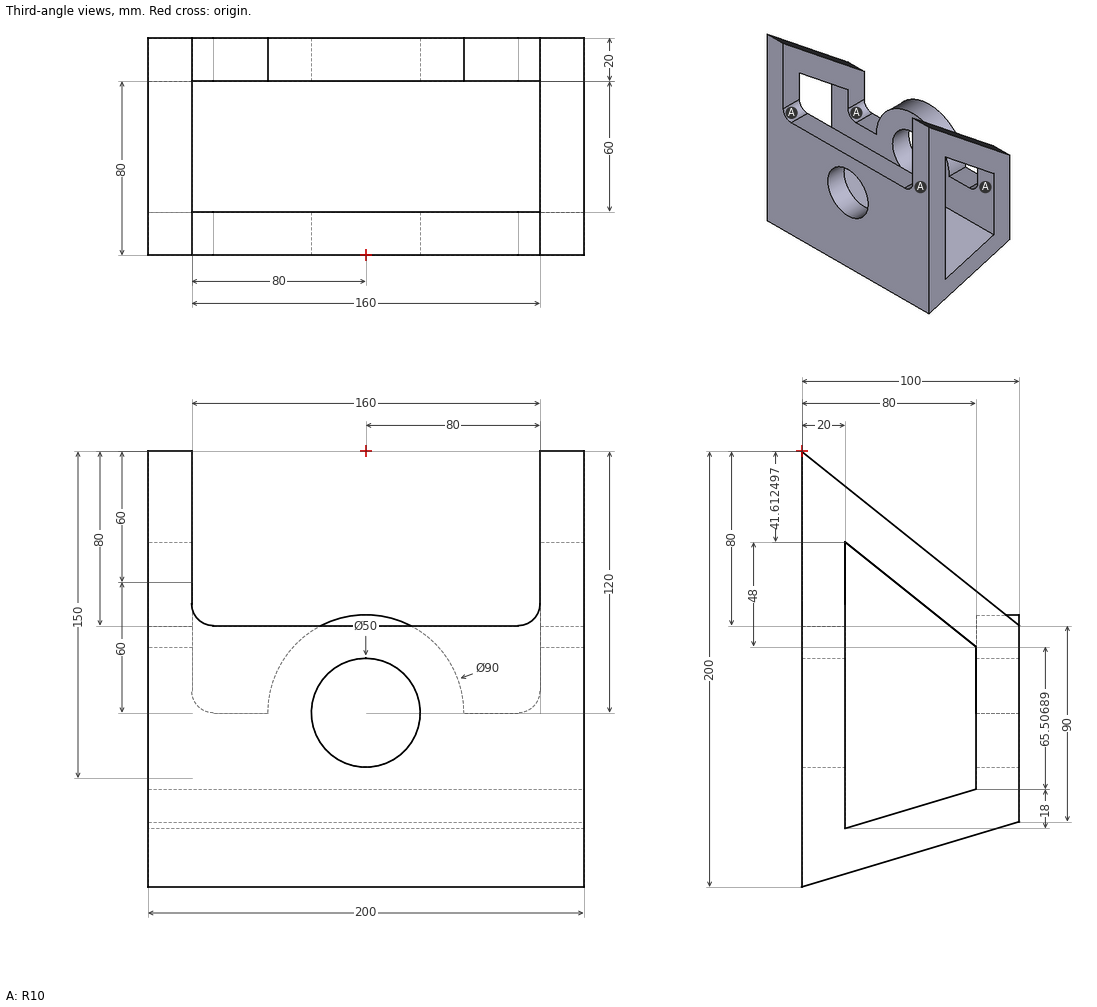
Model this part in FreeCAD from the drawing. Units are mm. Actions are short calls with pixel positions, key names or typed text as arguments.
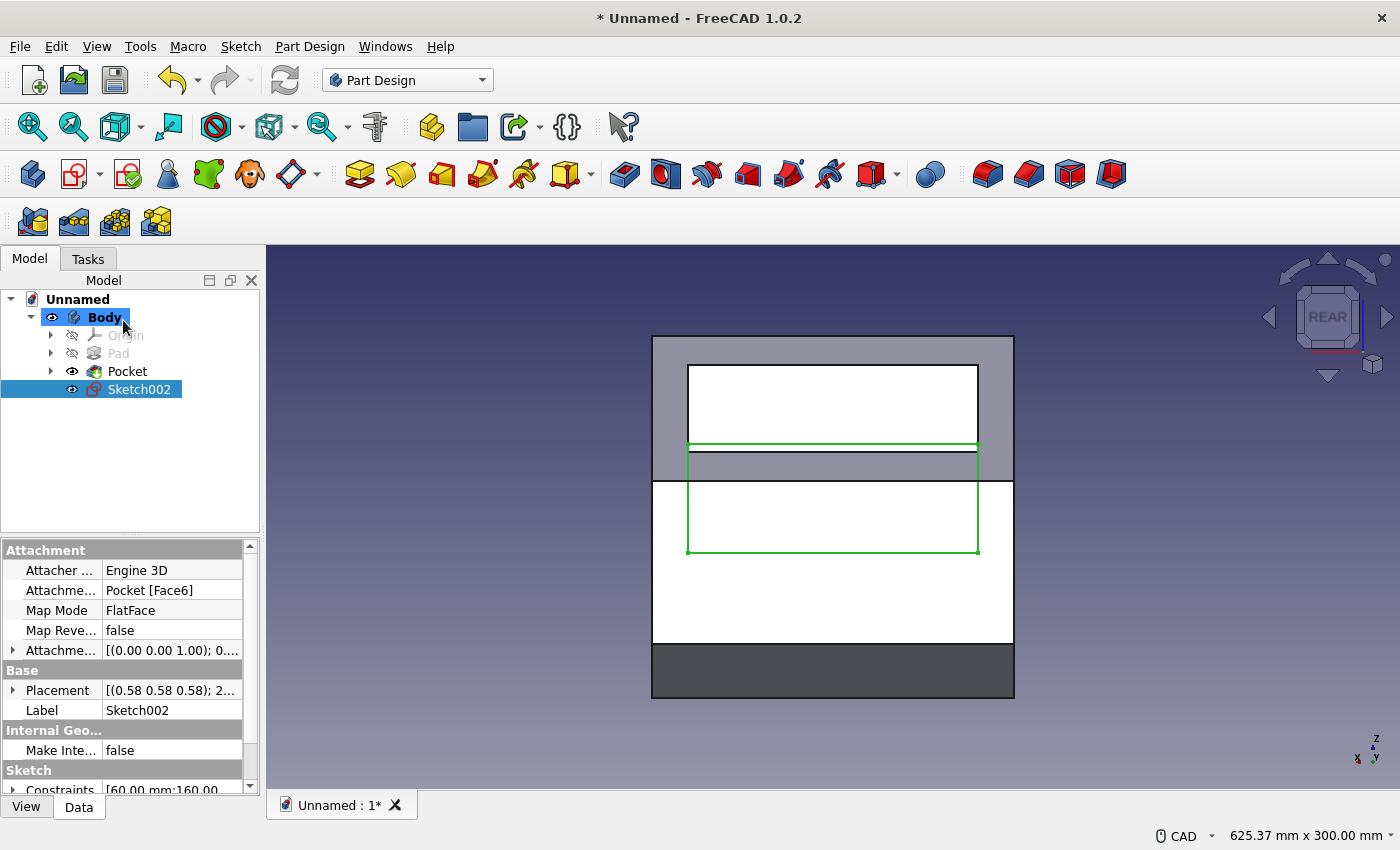
click(625, 174)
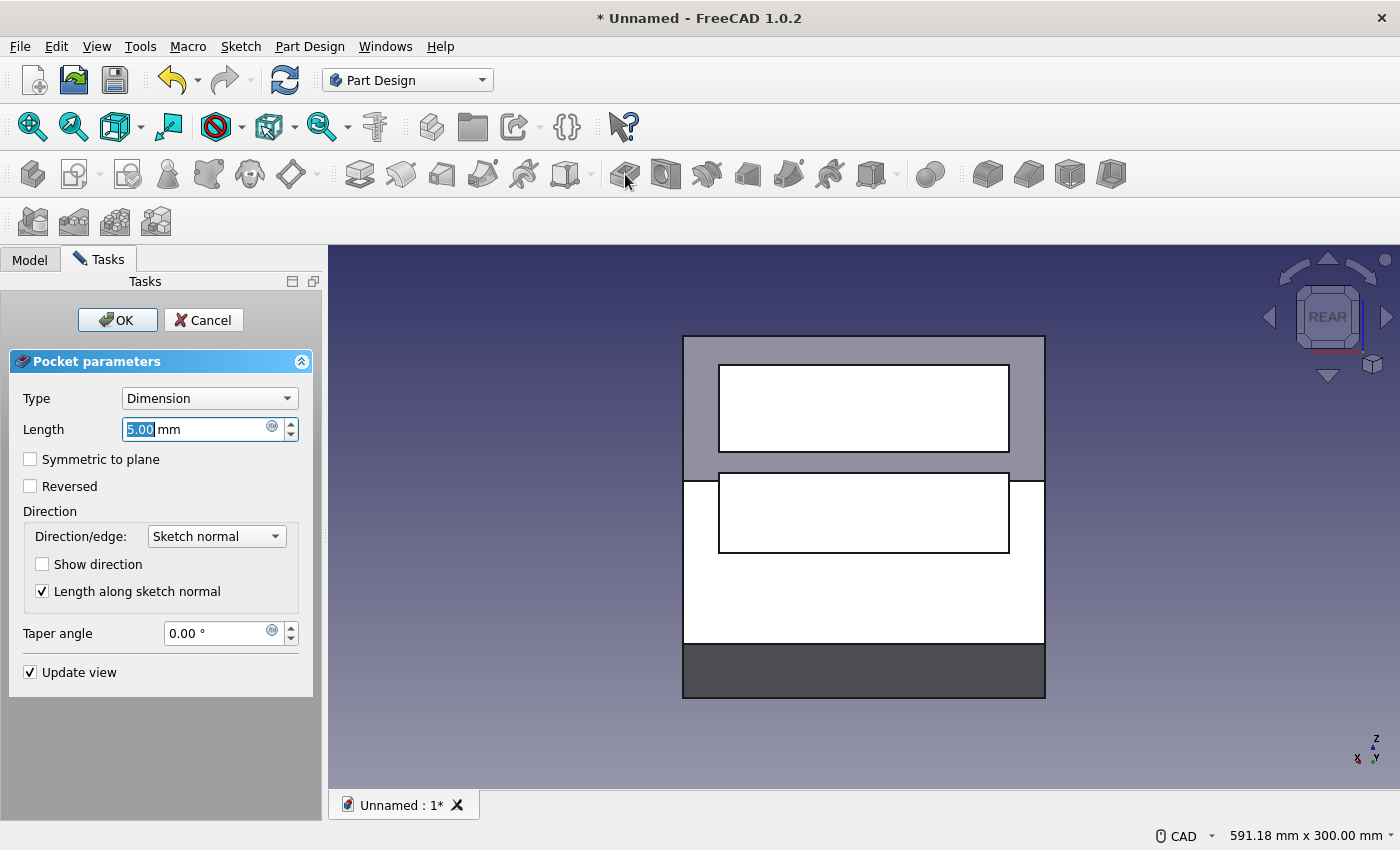
click(210, 398)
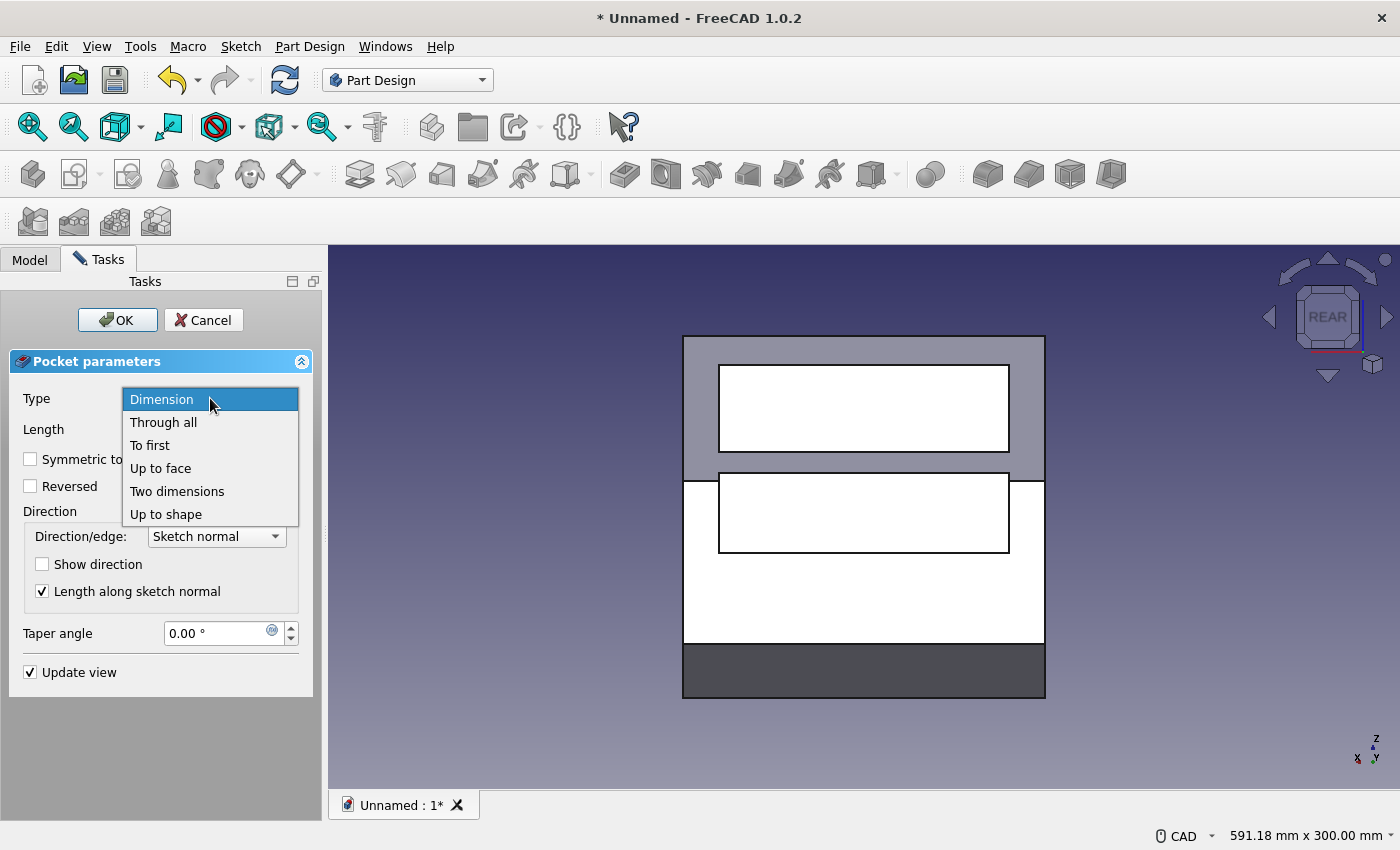
click(208, 446)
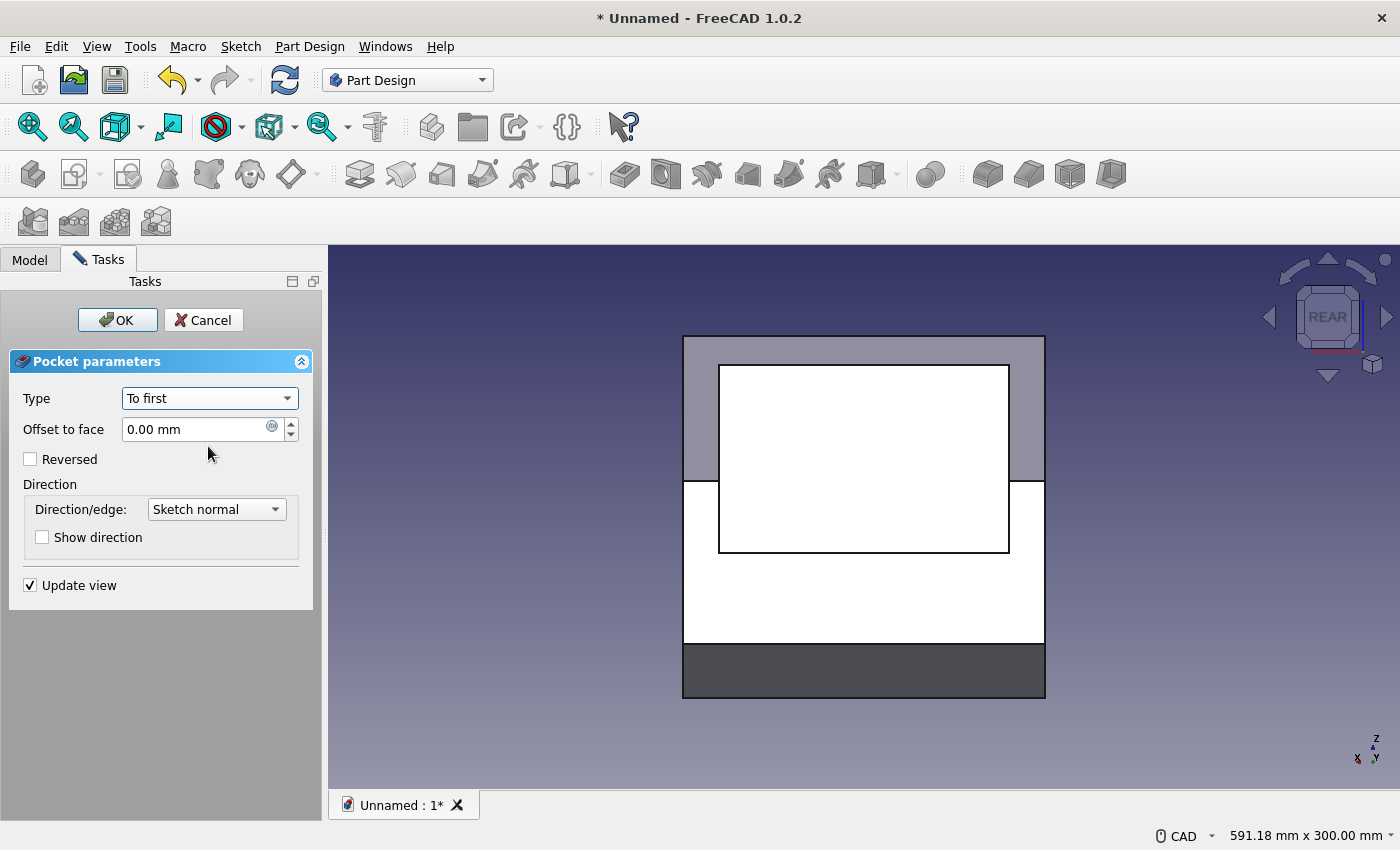
click(118, 320)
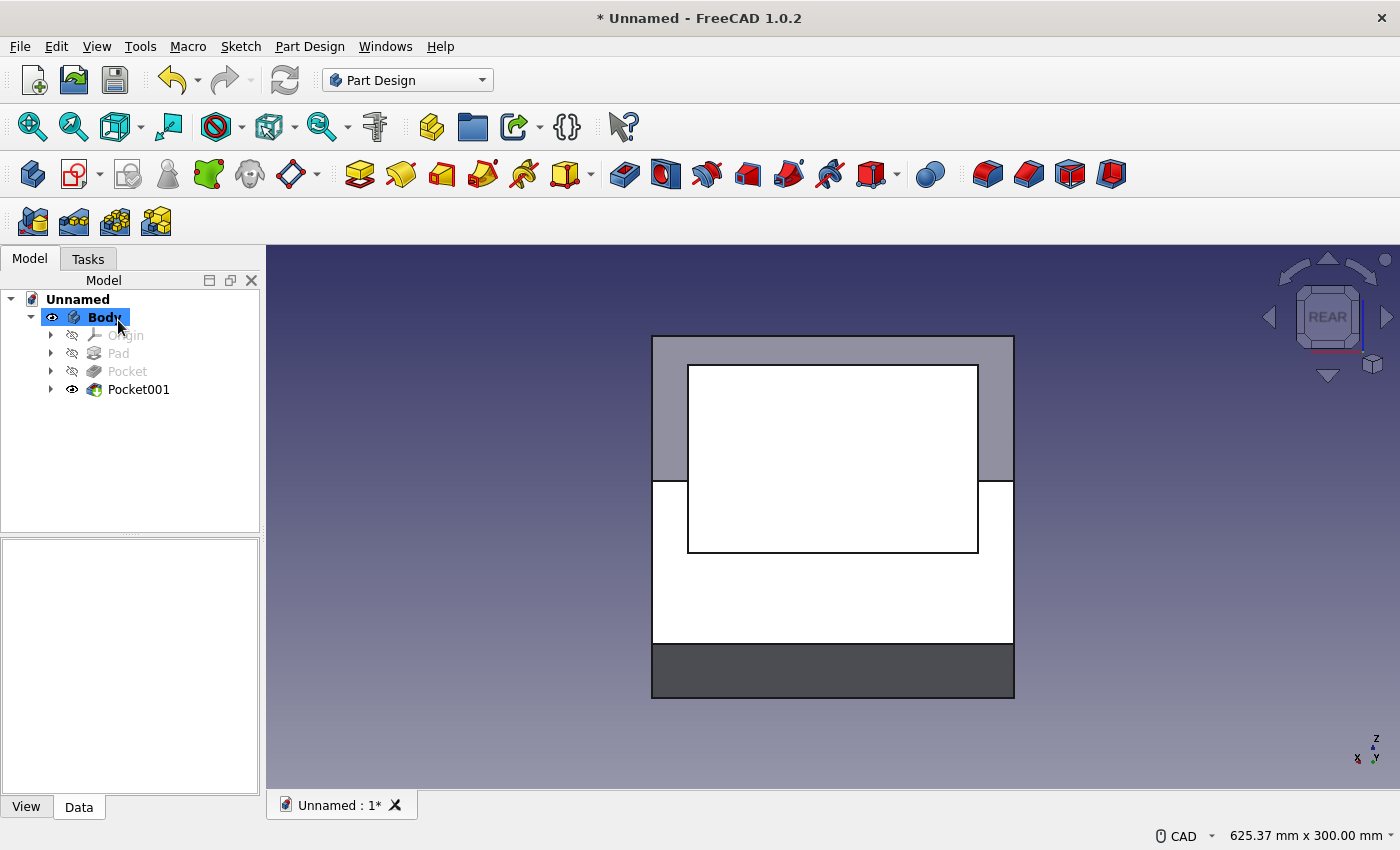
click(833, 506)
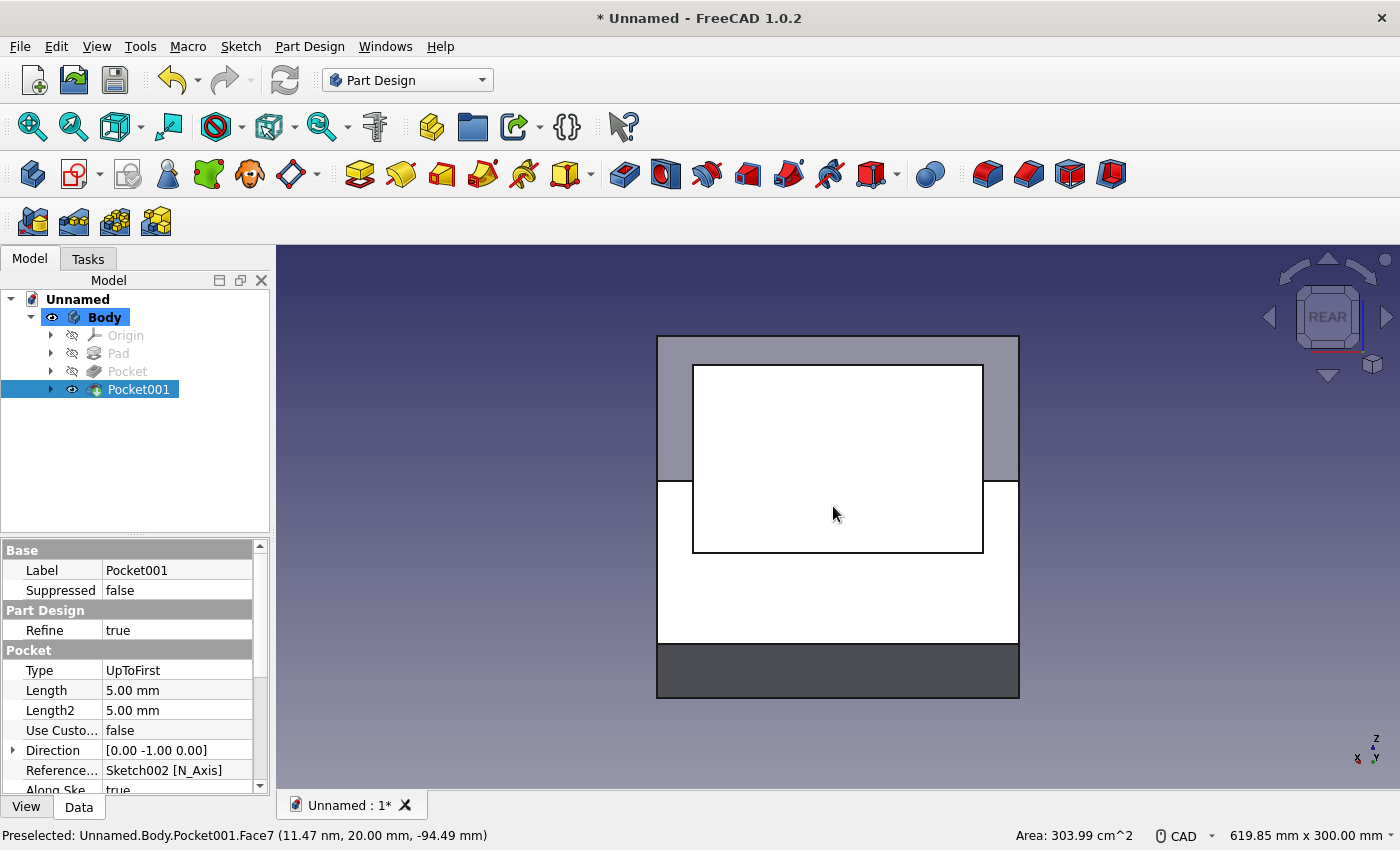
click(74, 174)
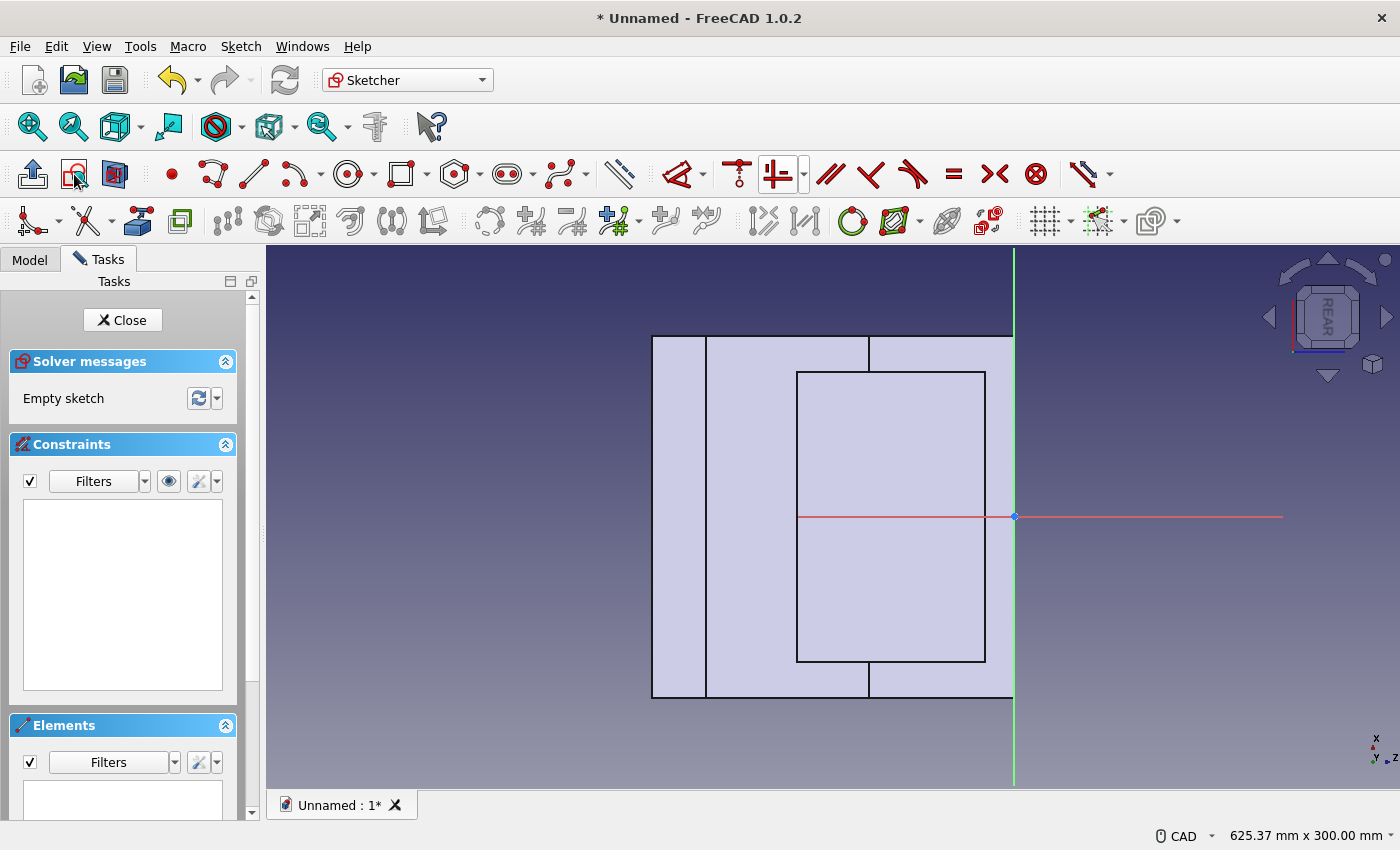
click(115, 174)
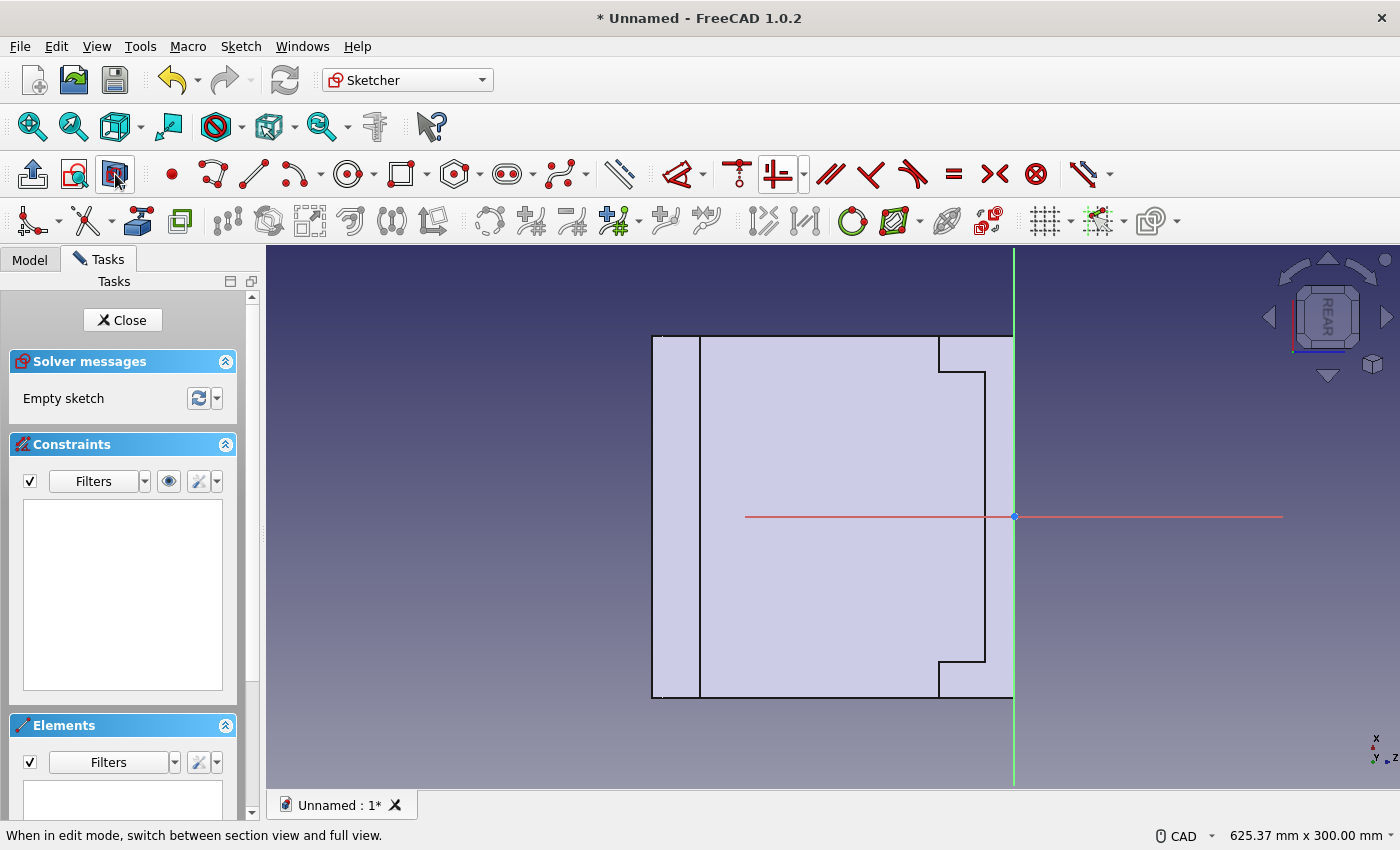
key(g)
key(r)